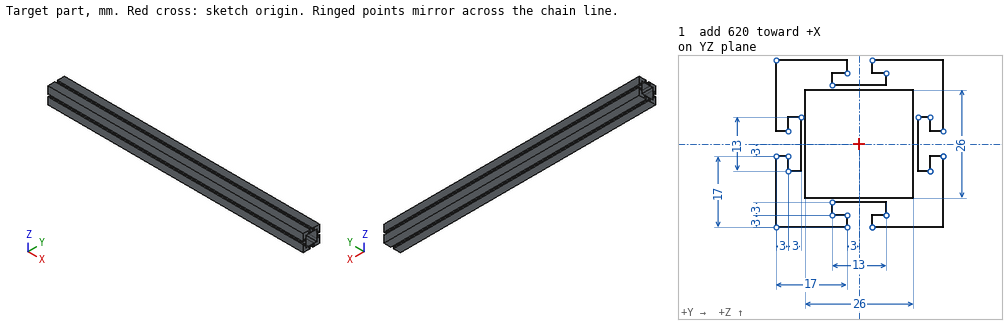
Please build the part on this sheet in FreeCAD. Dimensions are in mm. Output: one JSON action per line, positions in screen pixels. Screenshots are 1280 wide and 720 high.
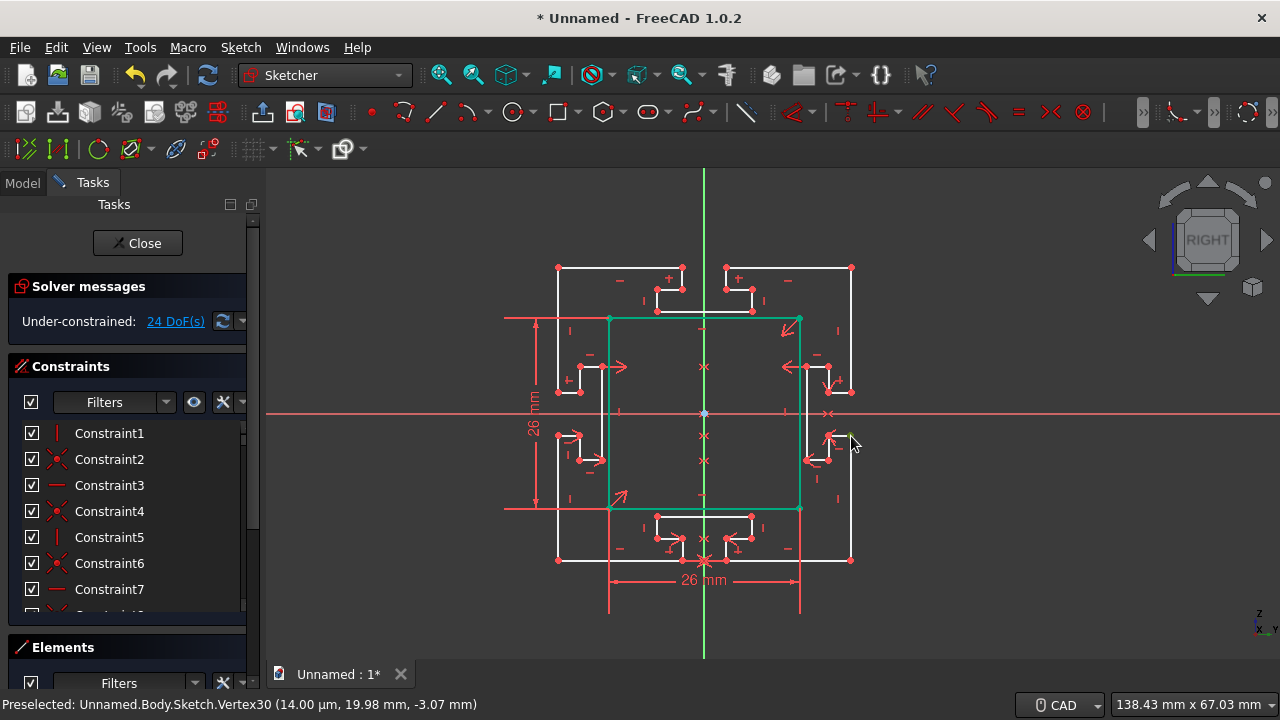
{"action": "left_click", "coordinate": [851, 393]}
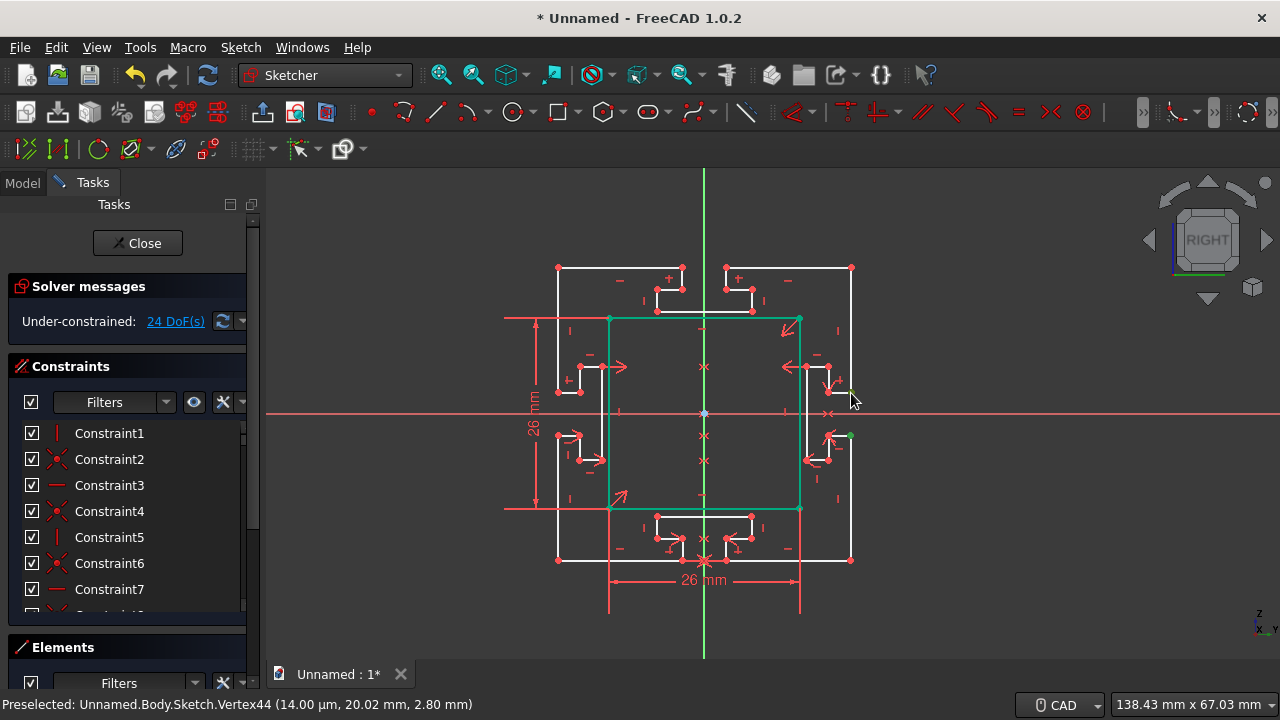
{"action": "left_click", "coordinate": [353, 414]}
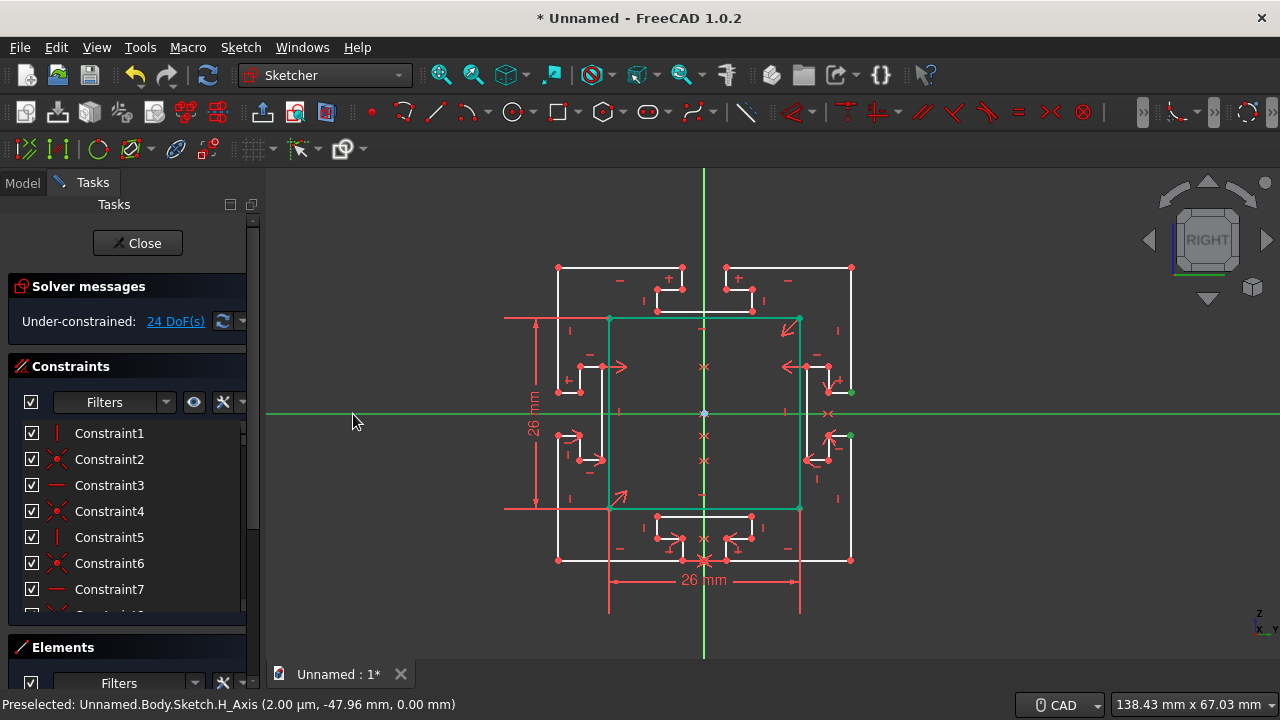
{"action": "key", "text": "s"}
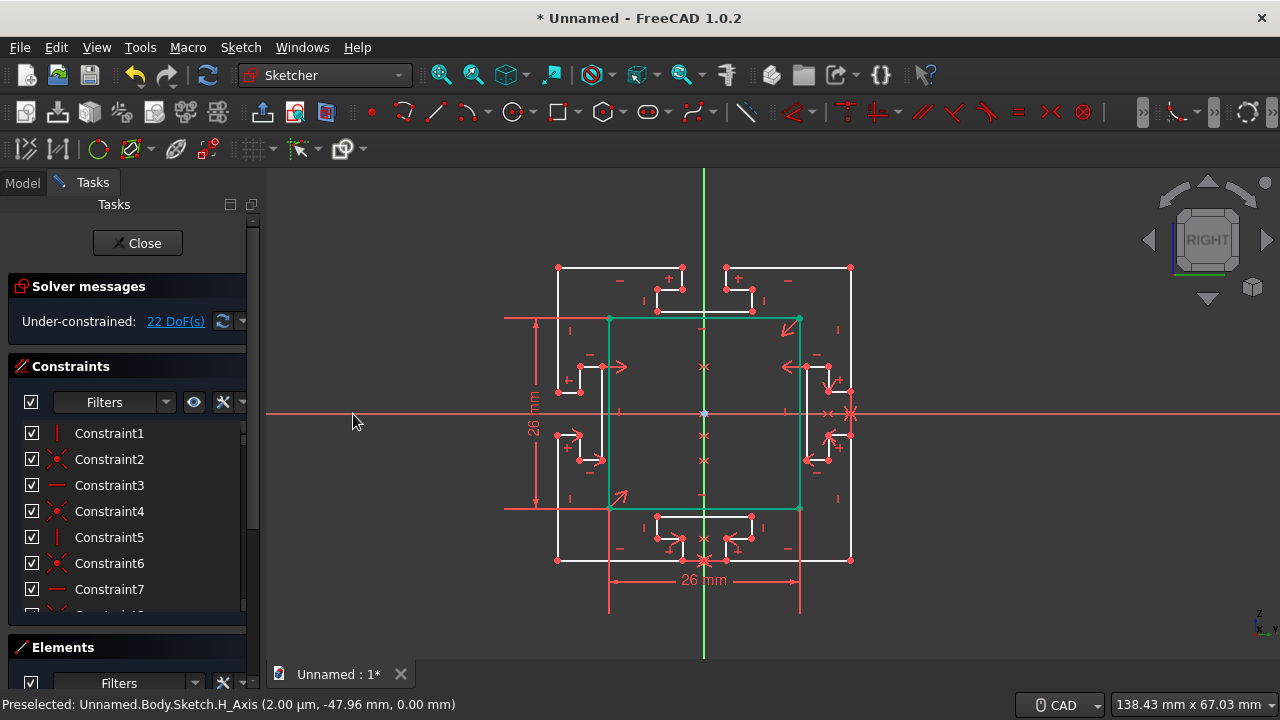
{"action": "left_click", "coordinate": [726, 561]}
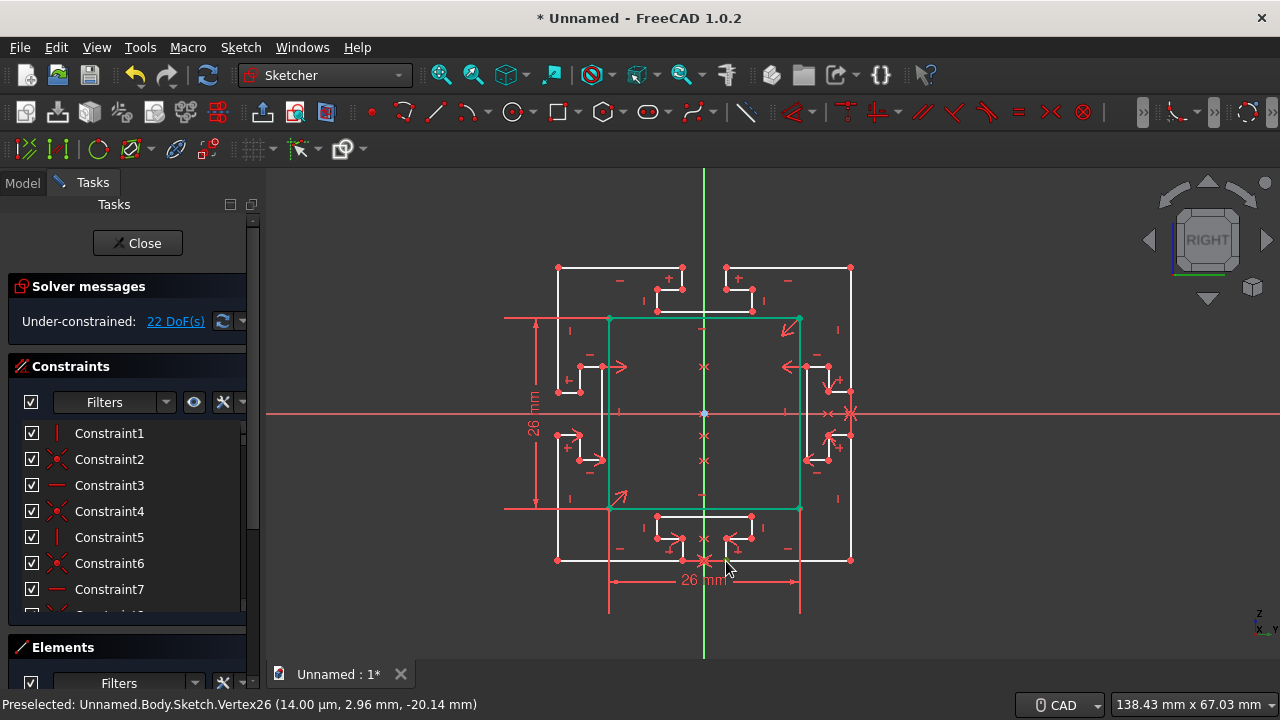
{"action": "left_click", "coordinate": [726, 268]}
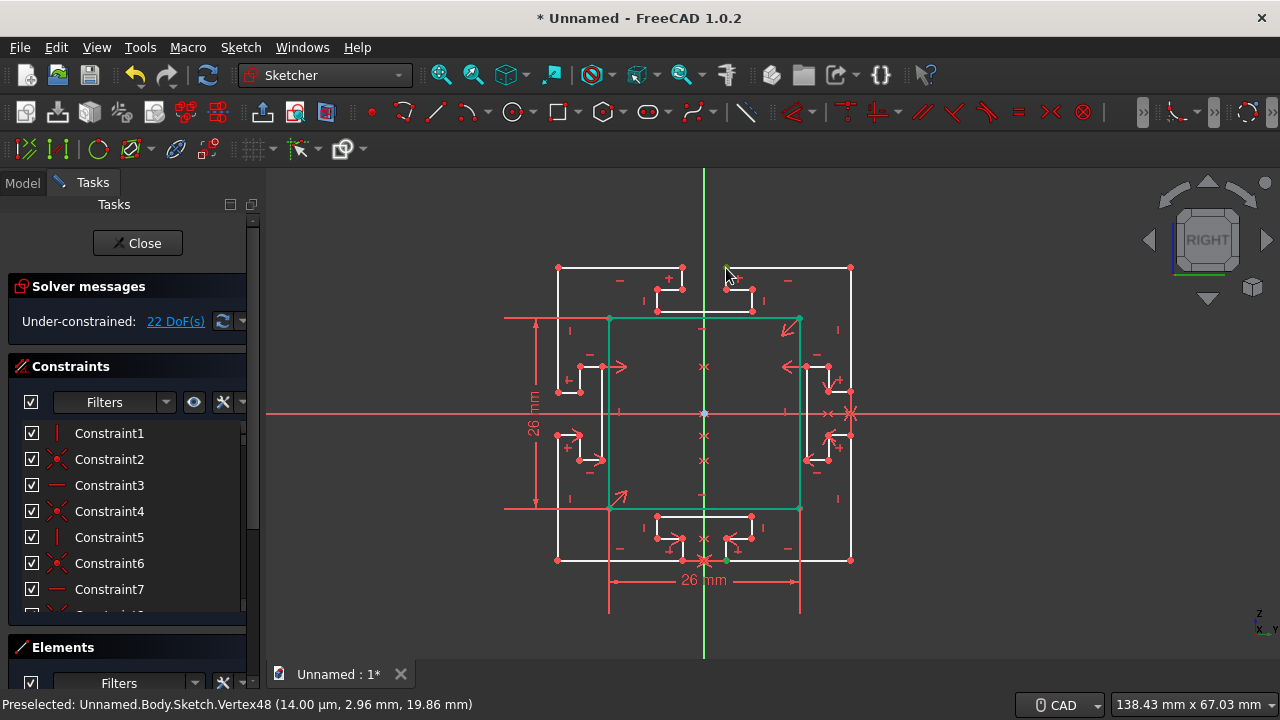
{"action": "left_click", "coordinate": [353, 414]}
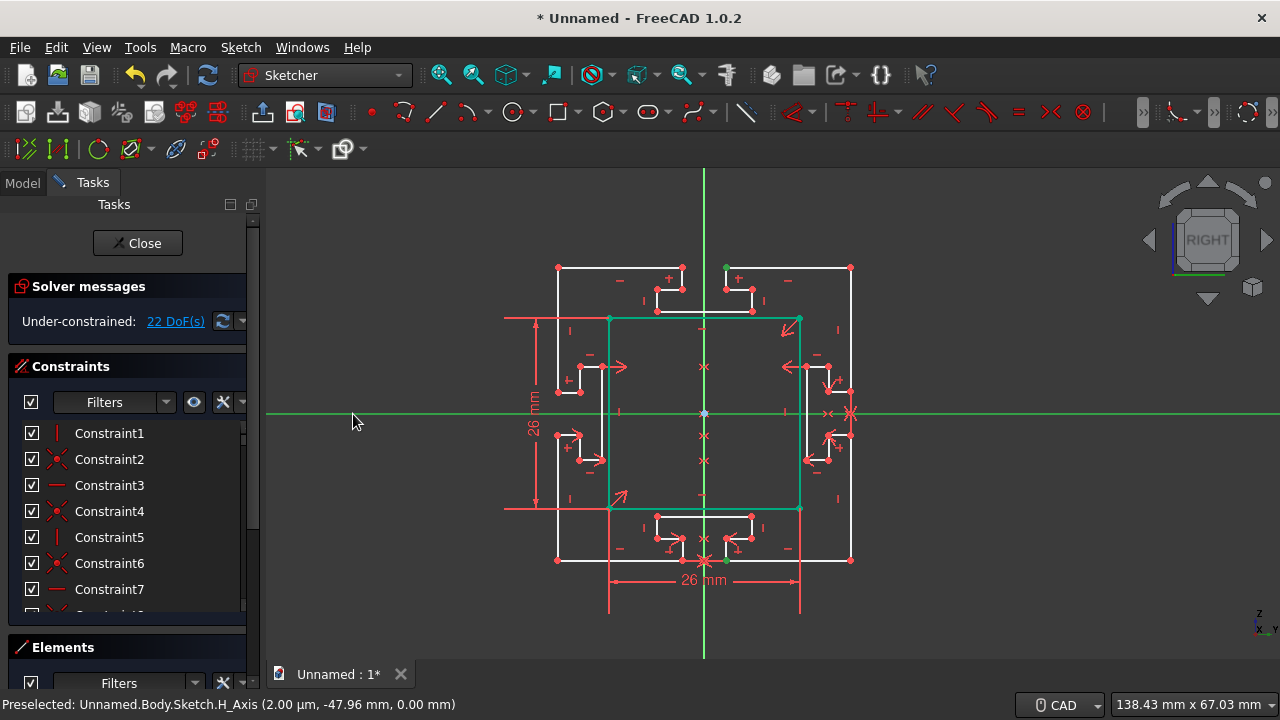
{"action": "key", "text": "s"}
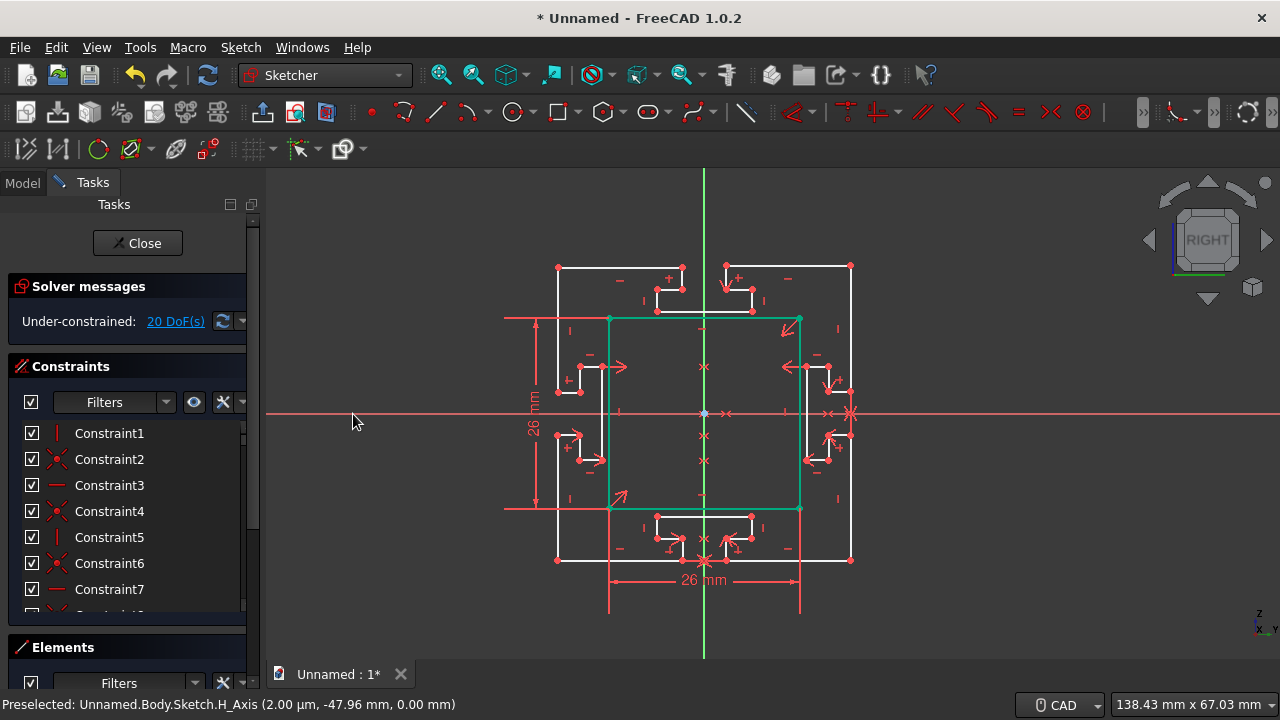
{"action": "left_click", "coordinate": [752, 539]}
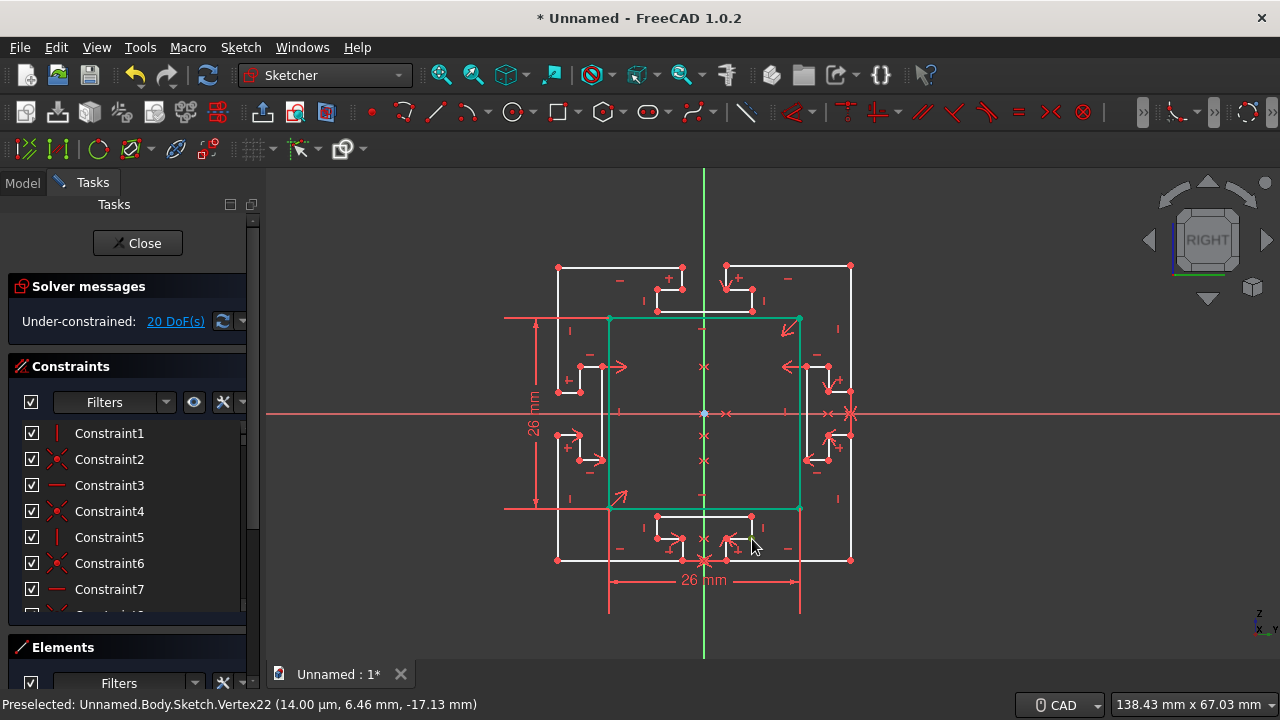
{"action": "left_click", "coordinate": [752, 290]}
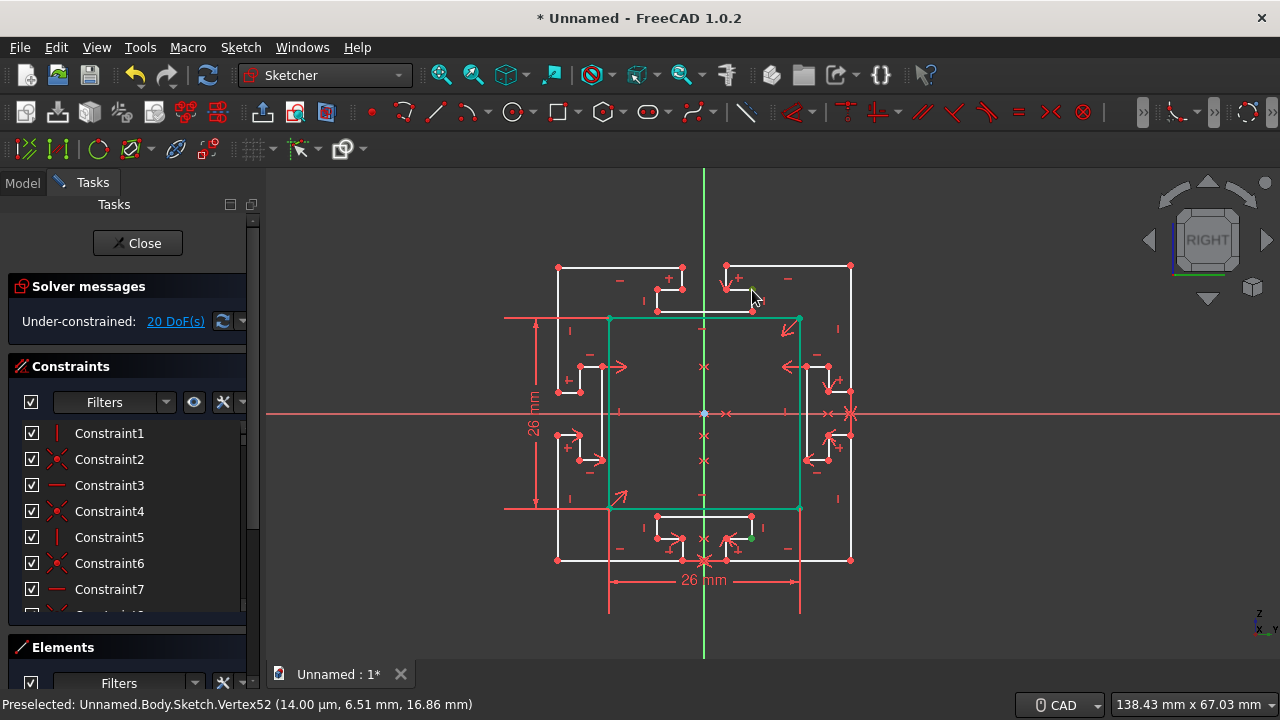
{"action": "left_click", "coordinate": [353, 414]}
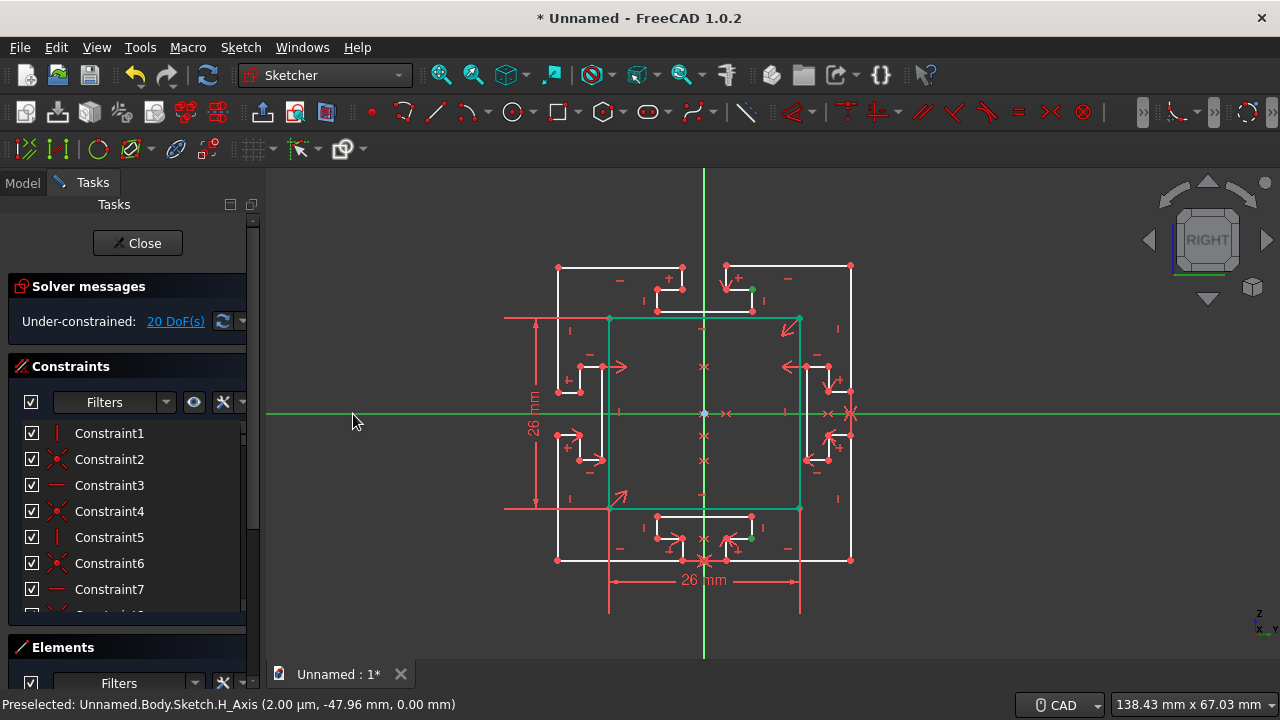
{"action": "key", "text": "s"}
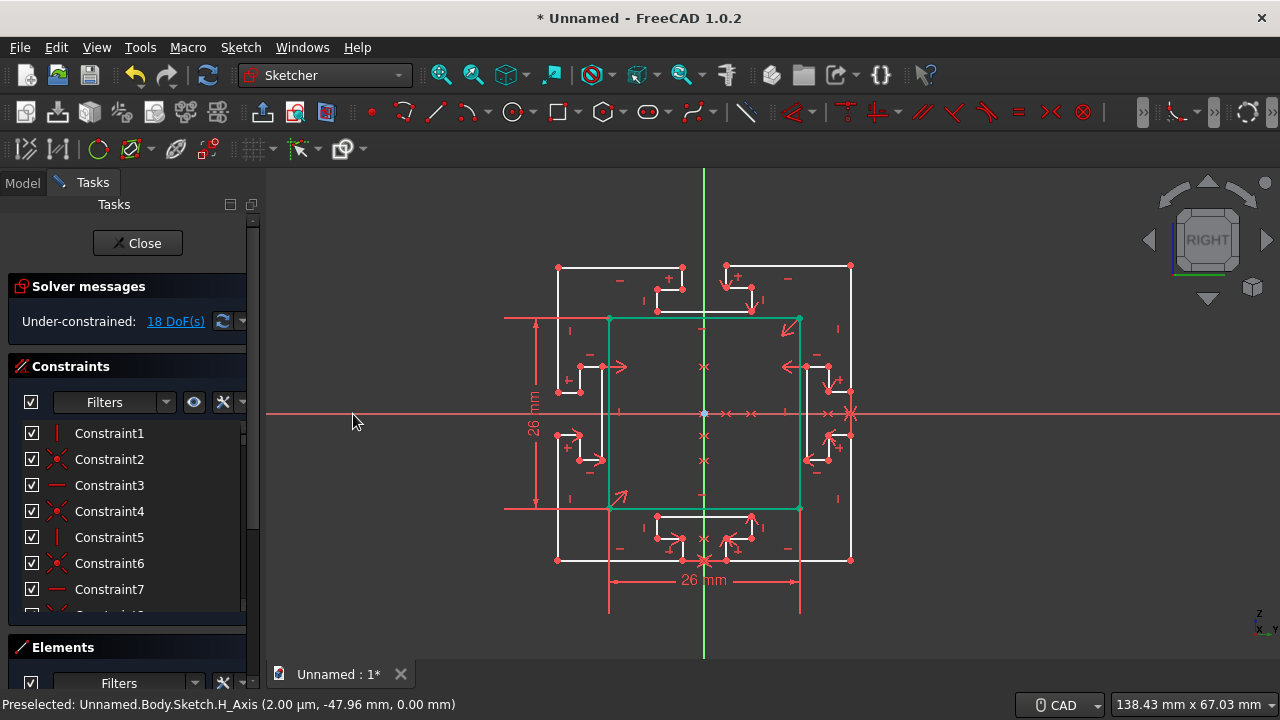
{"action": "left_click", "coordinate": [657, 517]}